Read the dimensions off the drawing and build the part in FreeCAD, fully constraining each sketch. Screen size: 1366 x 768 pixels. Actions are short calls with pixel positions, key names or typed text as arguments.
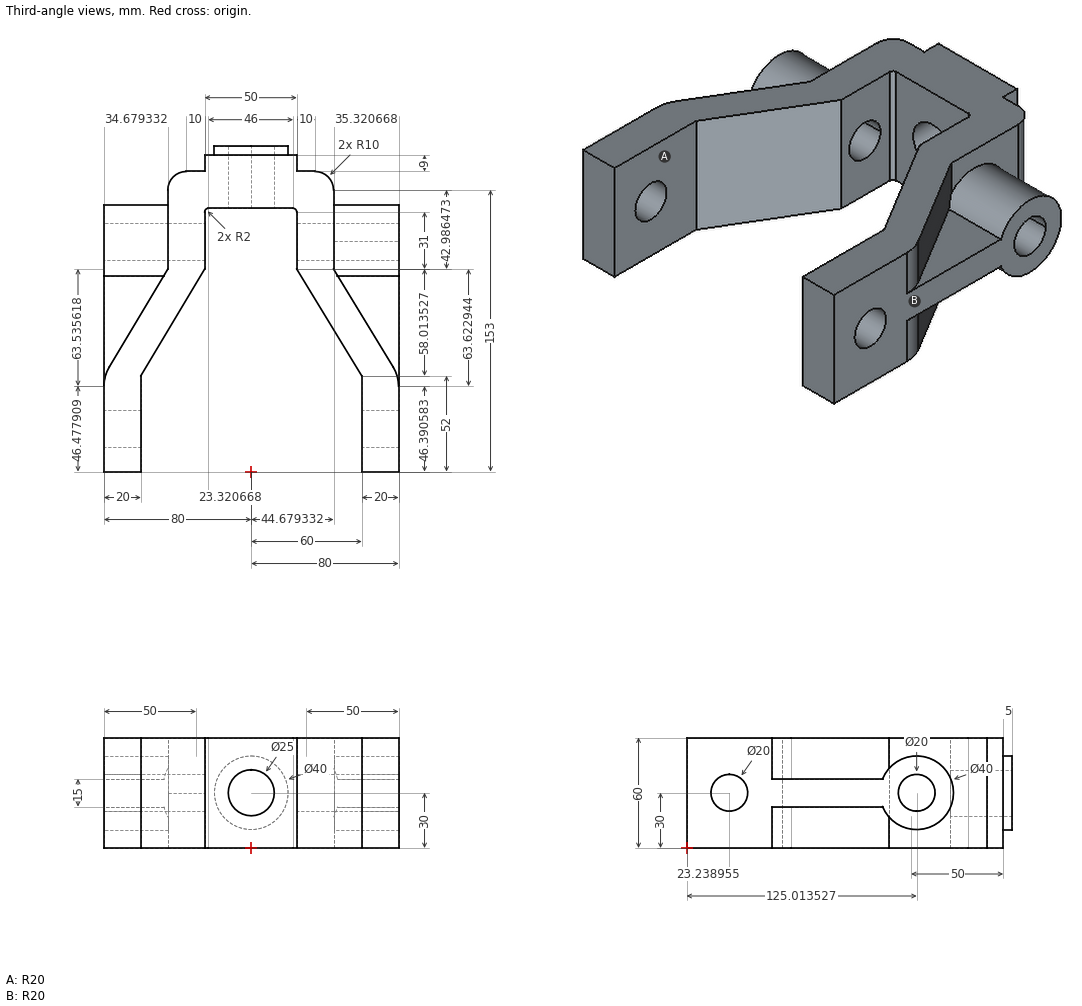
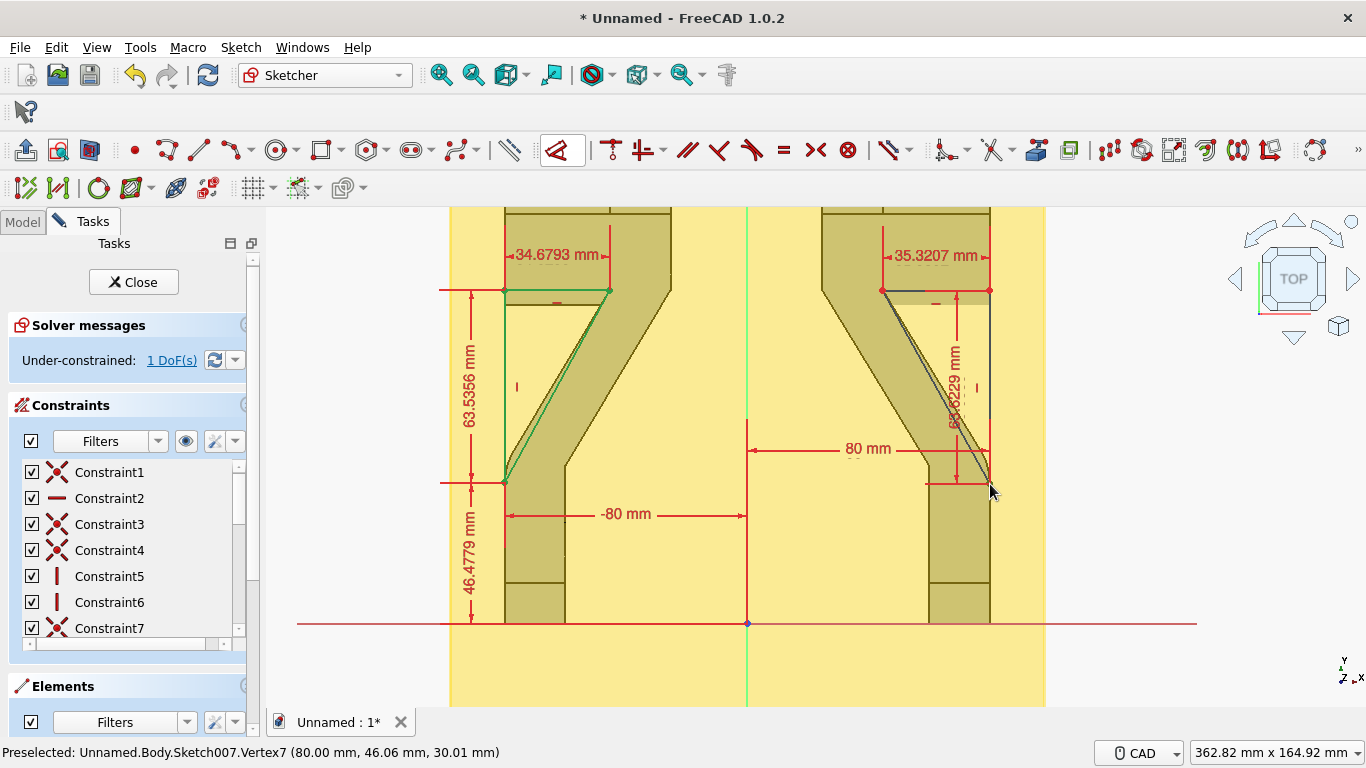
key(i)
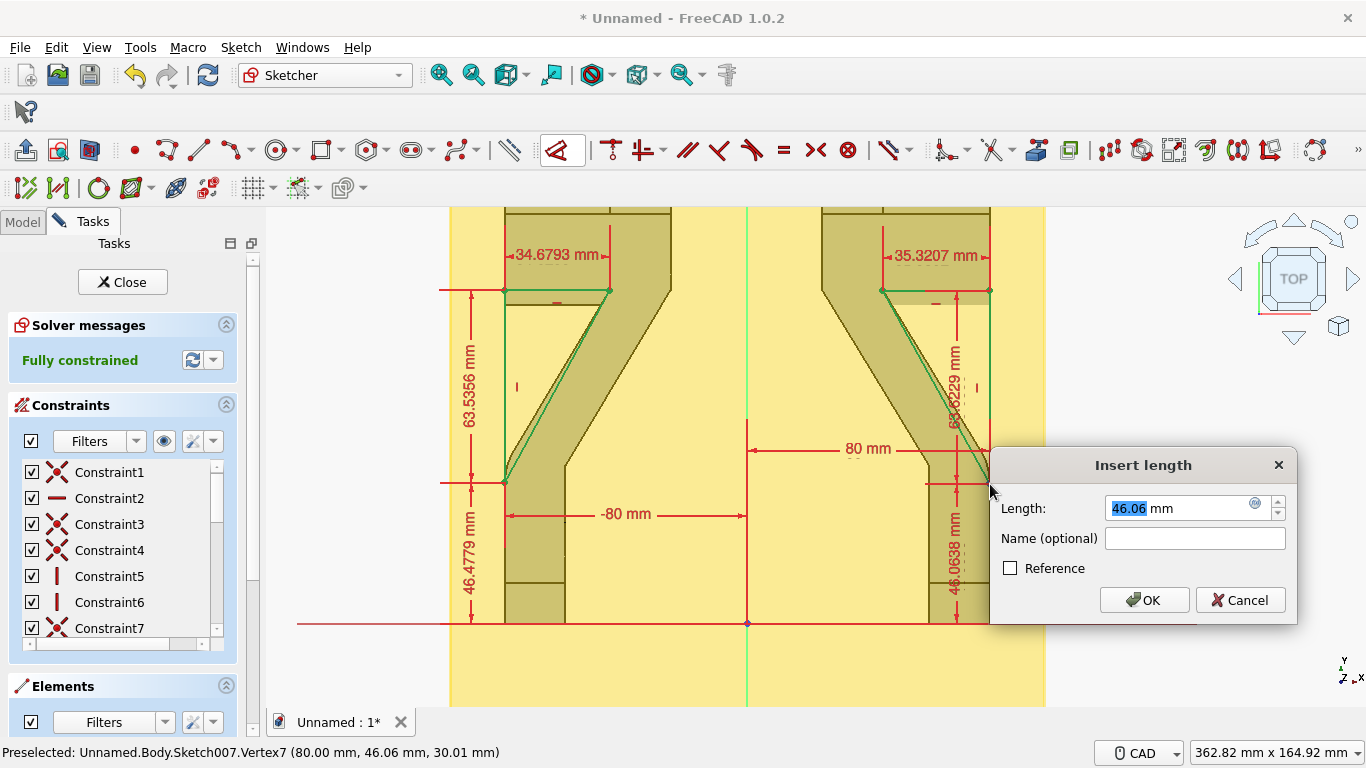
text(46.390583)
key(Return)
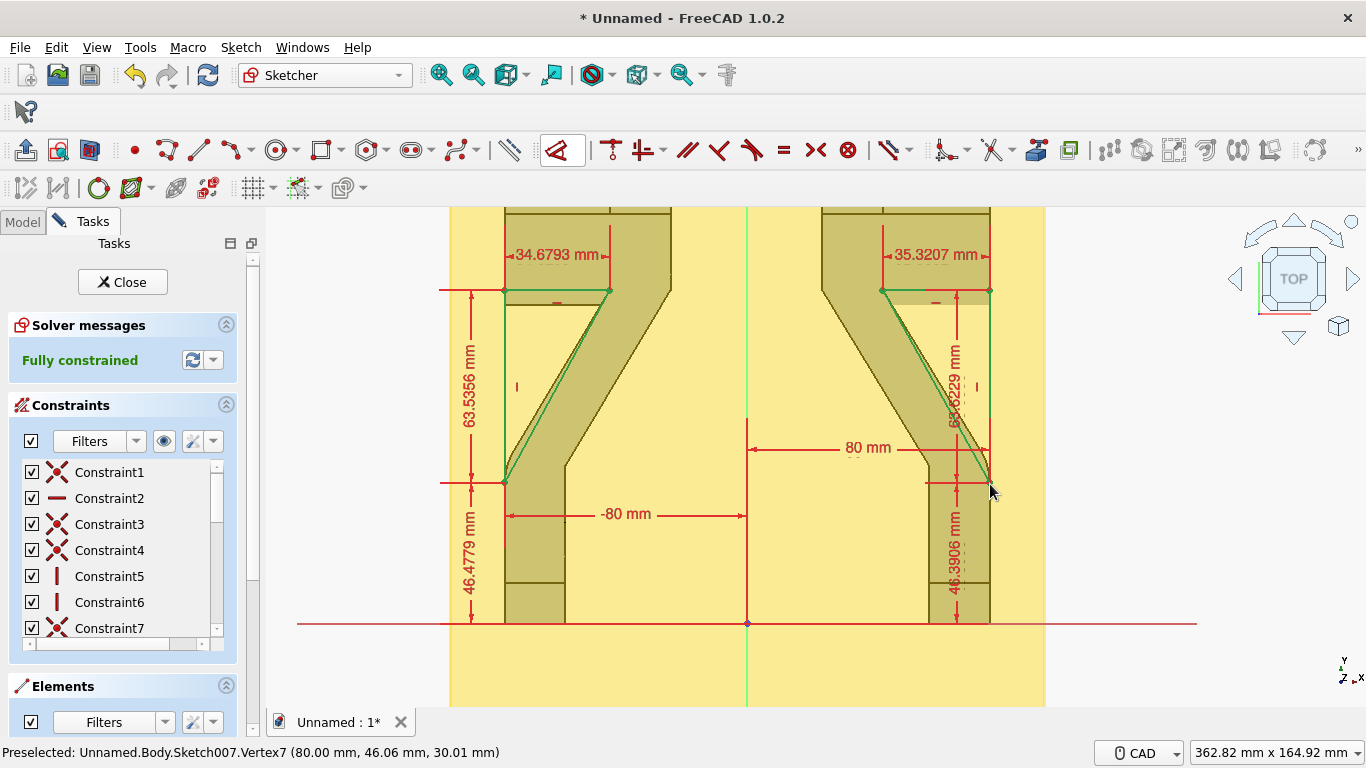
click(123, 282)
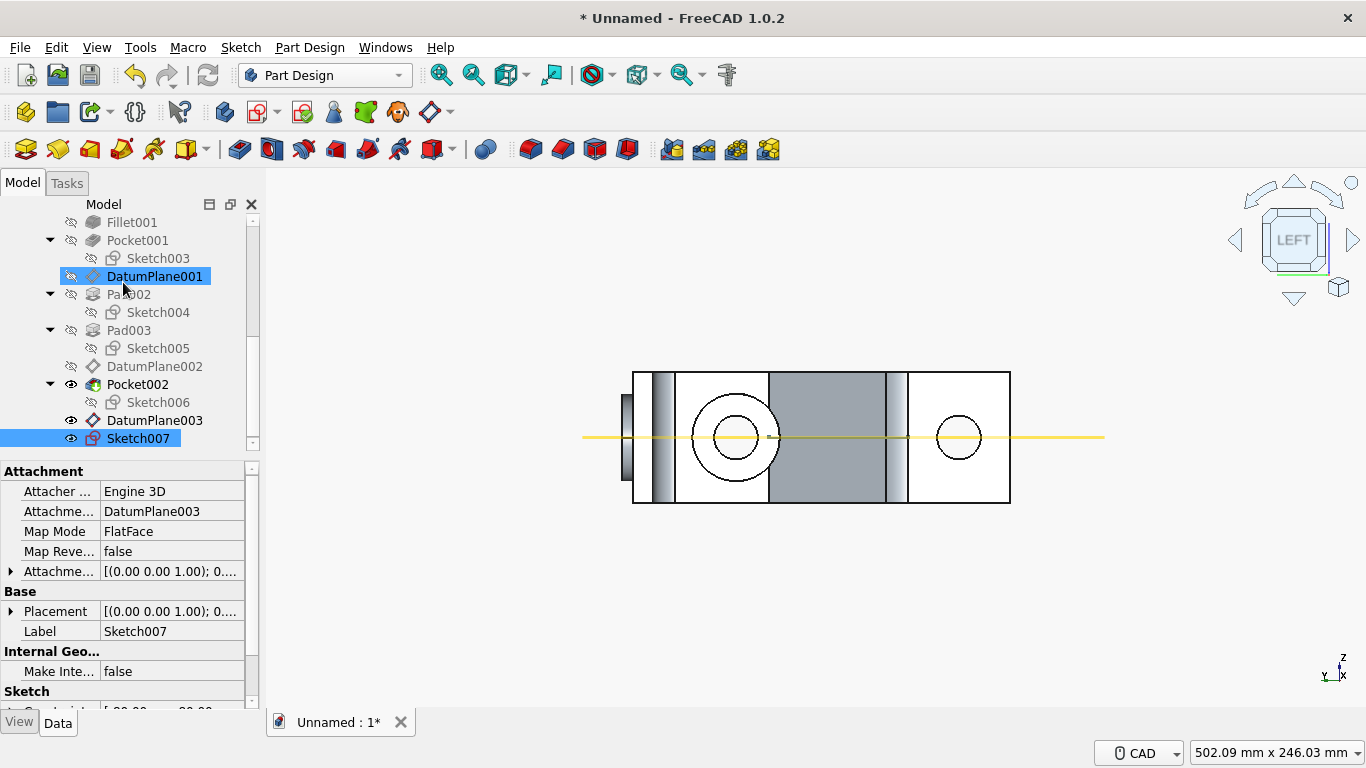
click(26, 150)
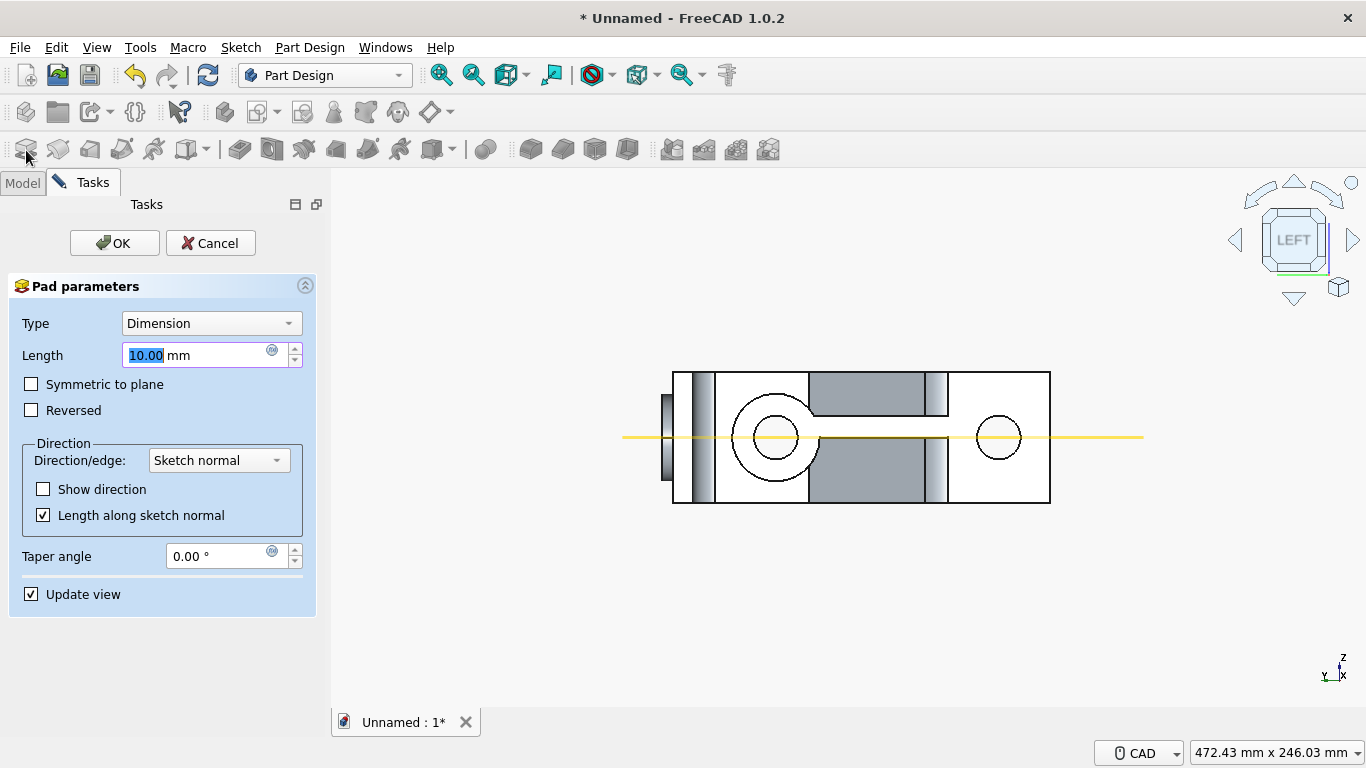
text(15)
key(Tab)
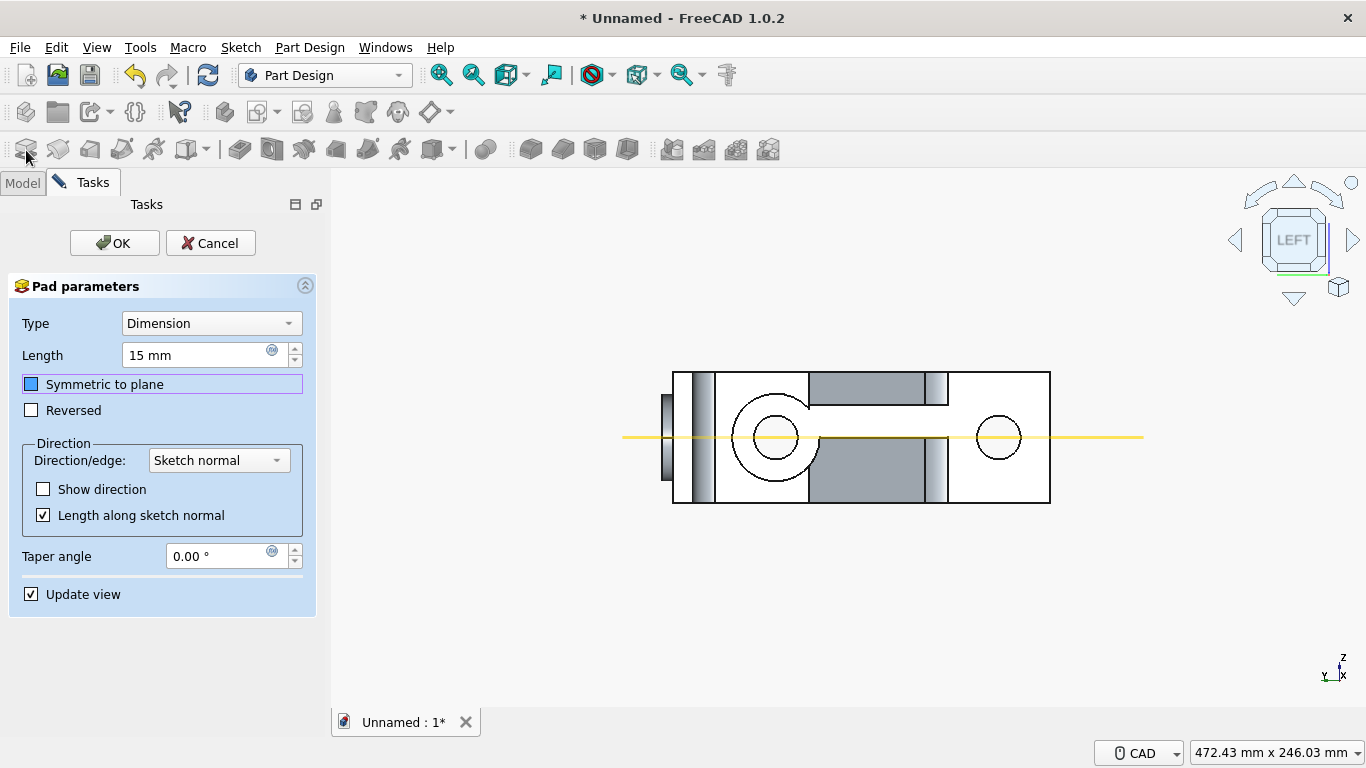
click(30, 384)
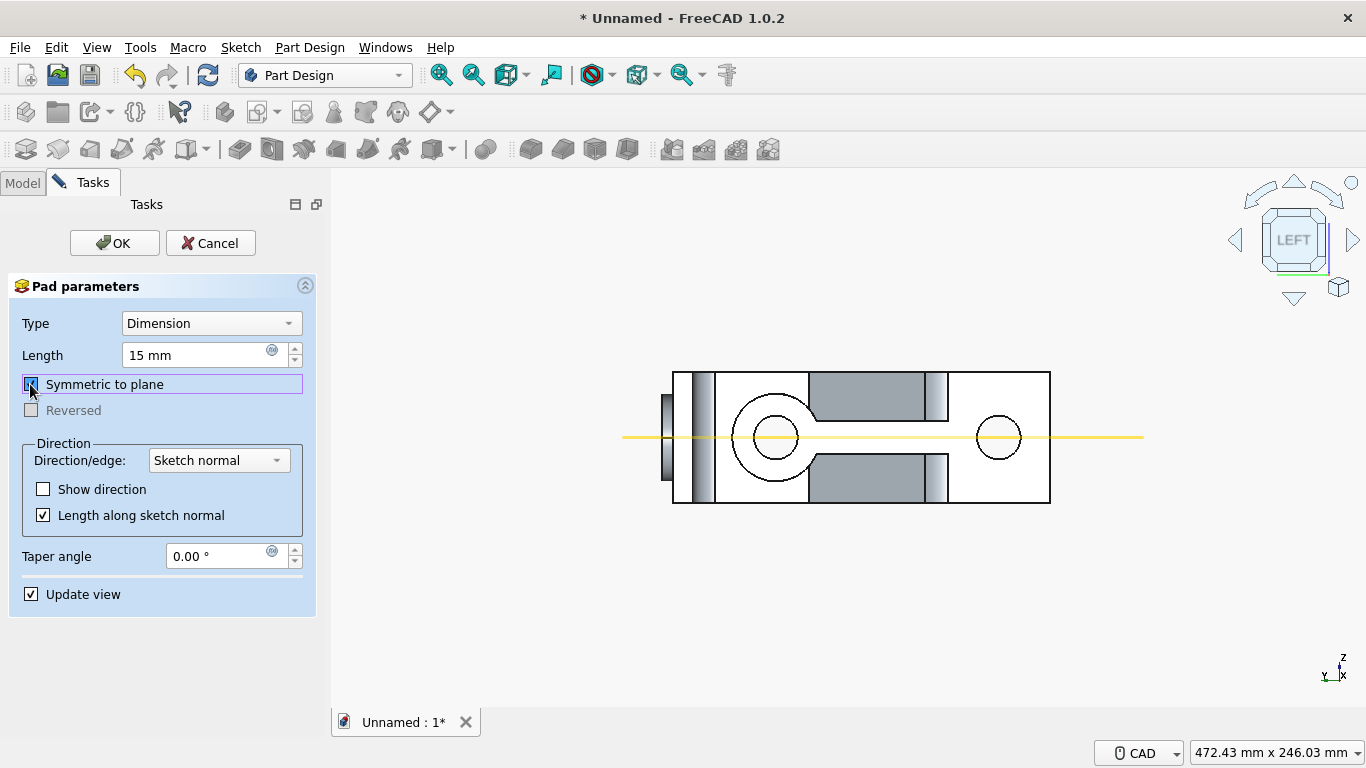
click(115, 243)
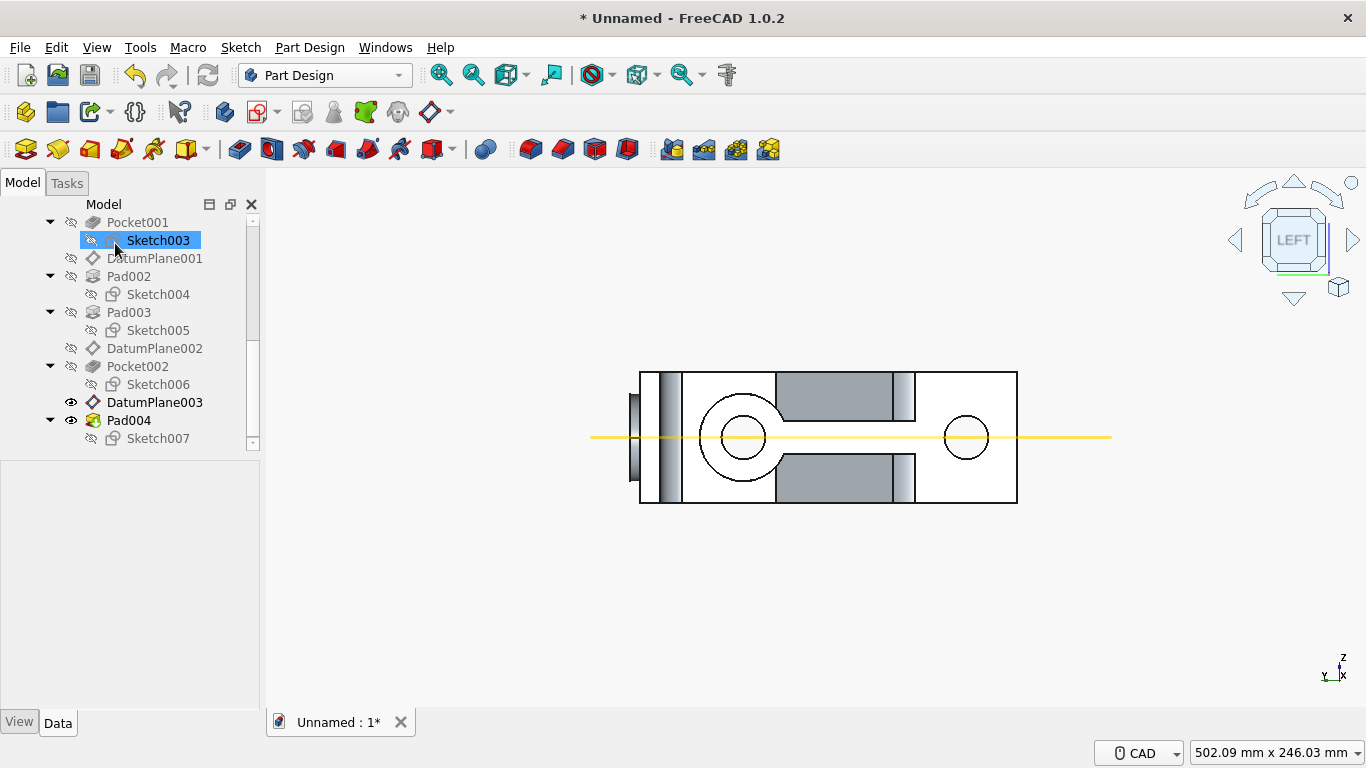
click(116, 402)
key(space)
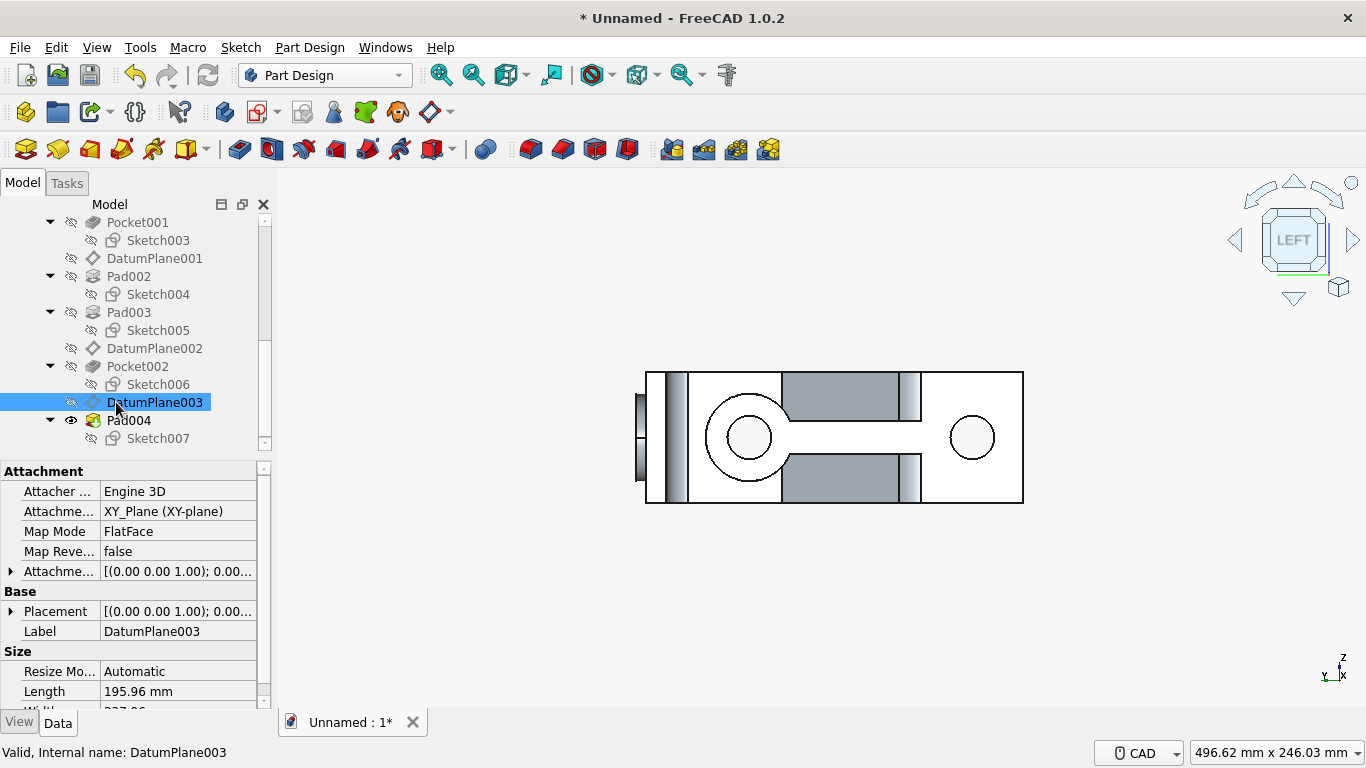
key(0)